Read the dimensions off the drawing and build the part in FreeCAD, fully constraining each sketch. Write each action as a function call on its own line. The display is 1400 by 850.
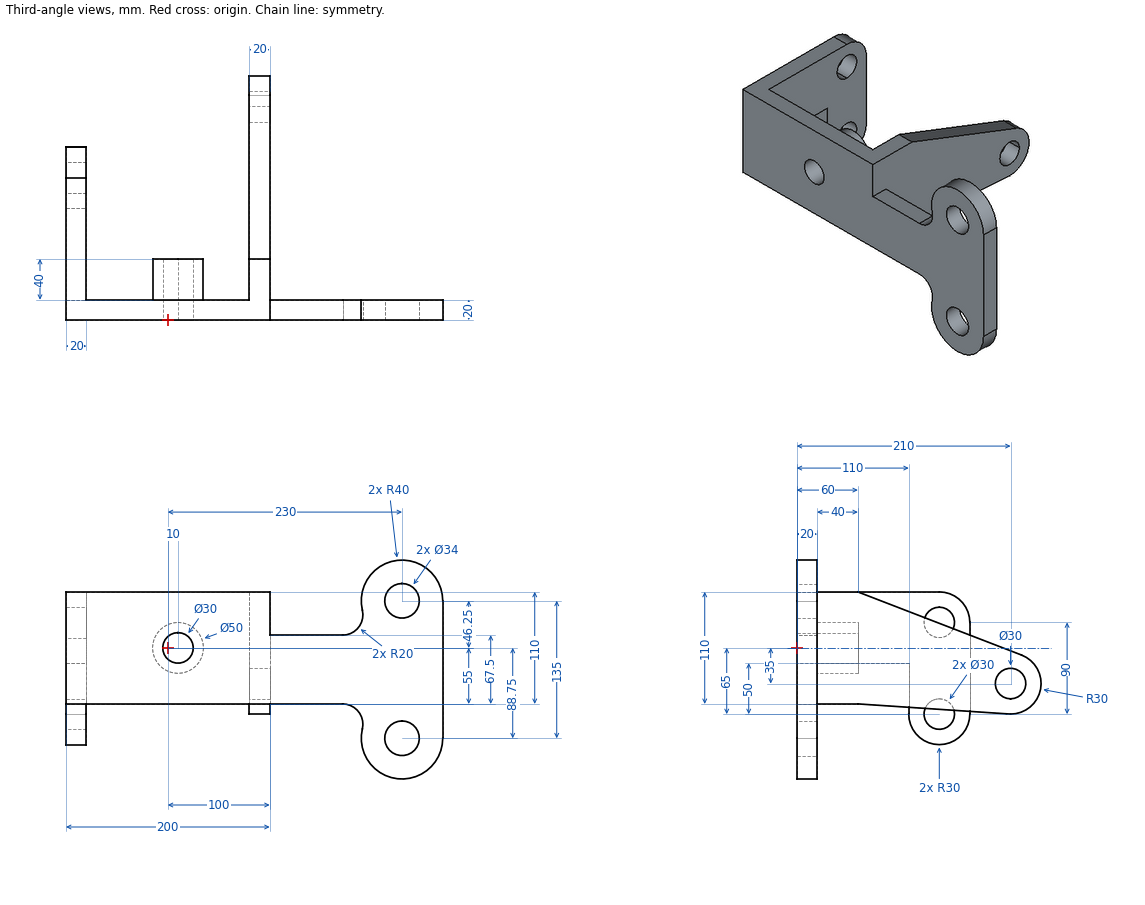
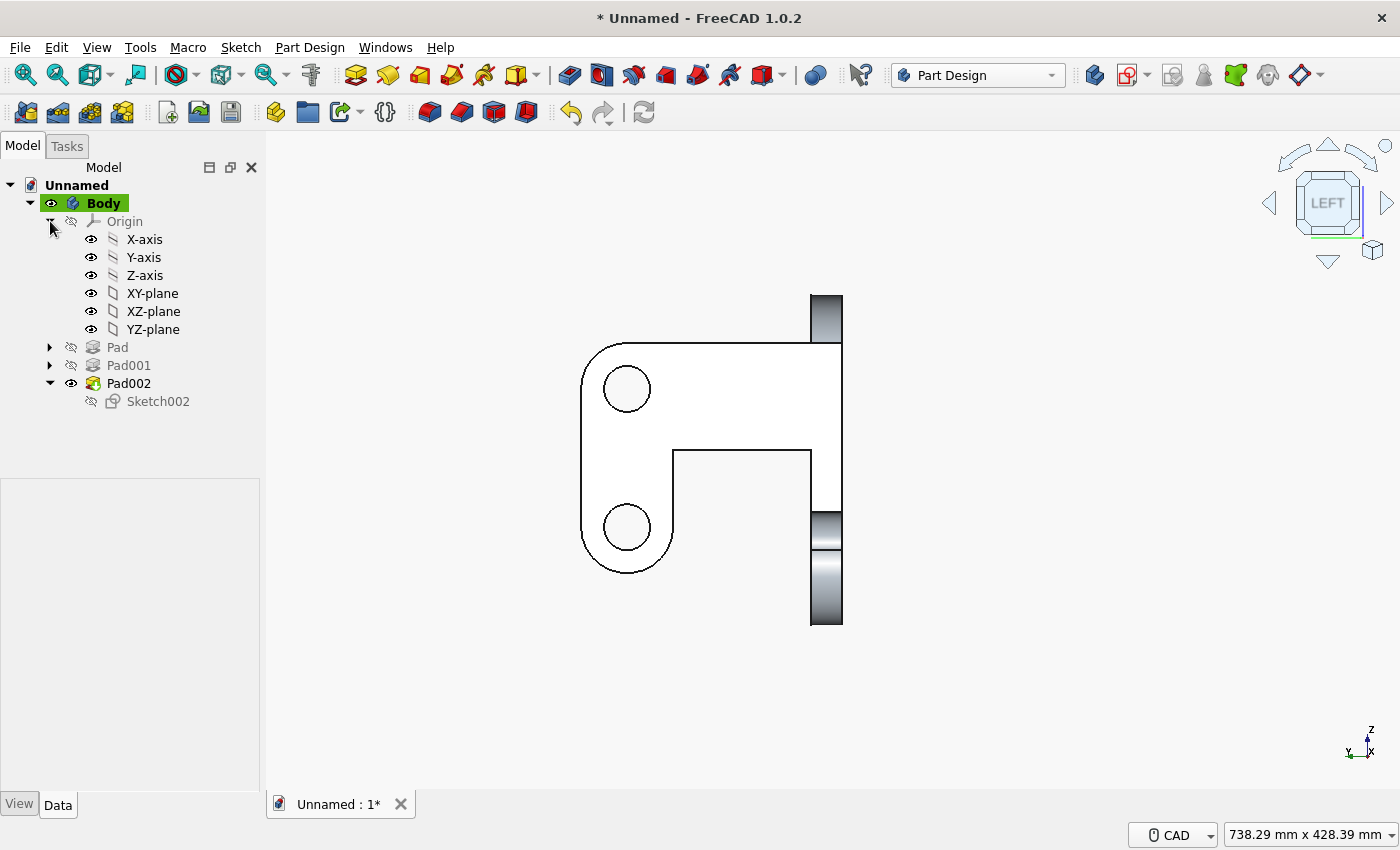
click(136, 329)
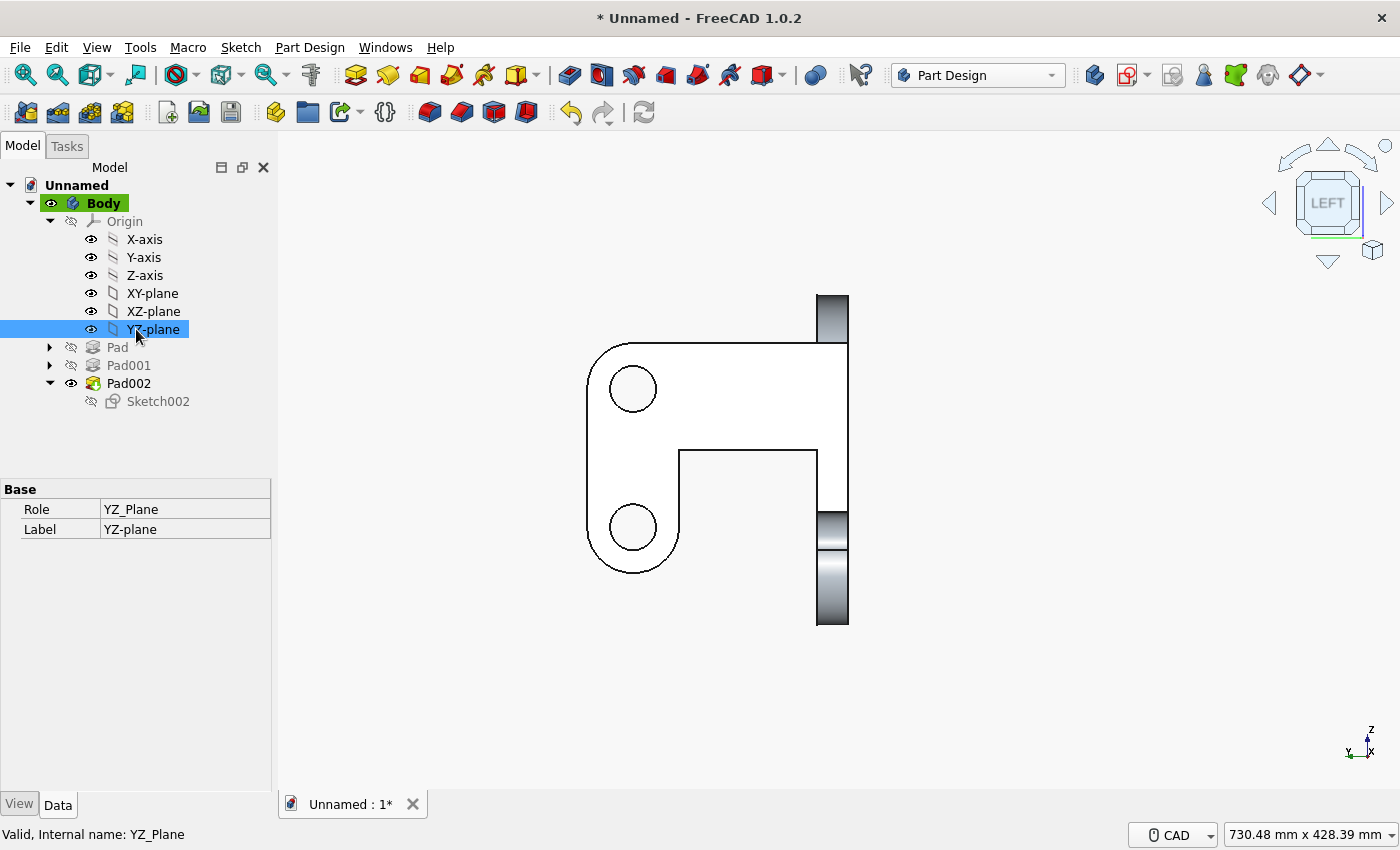
click(1300, 76)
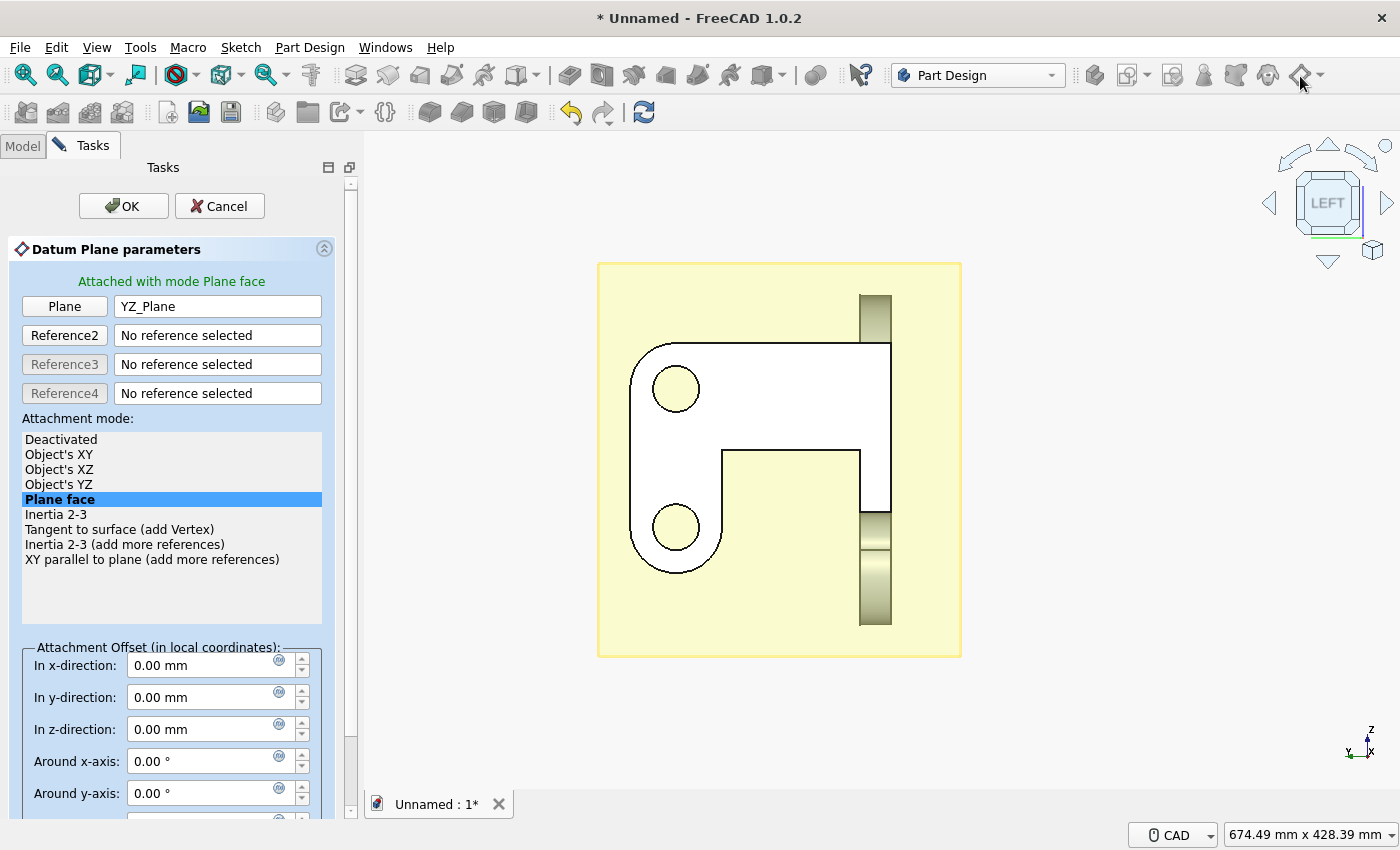
triple_click(210, 729)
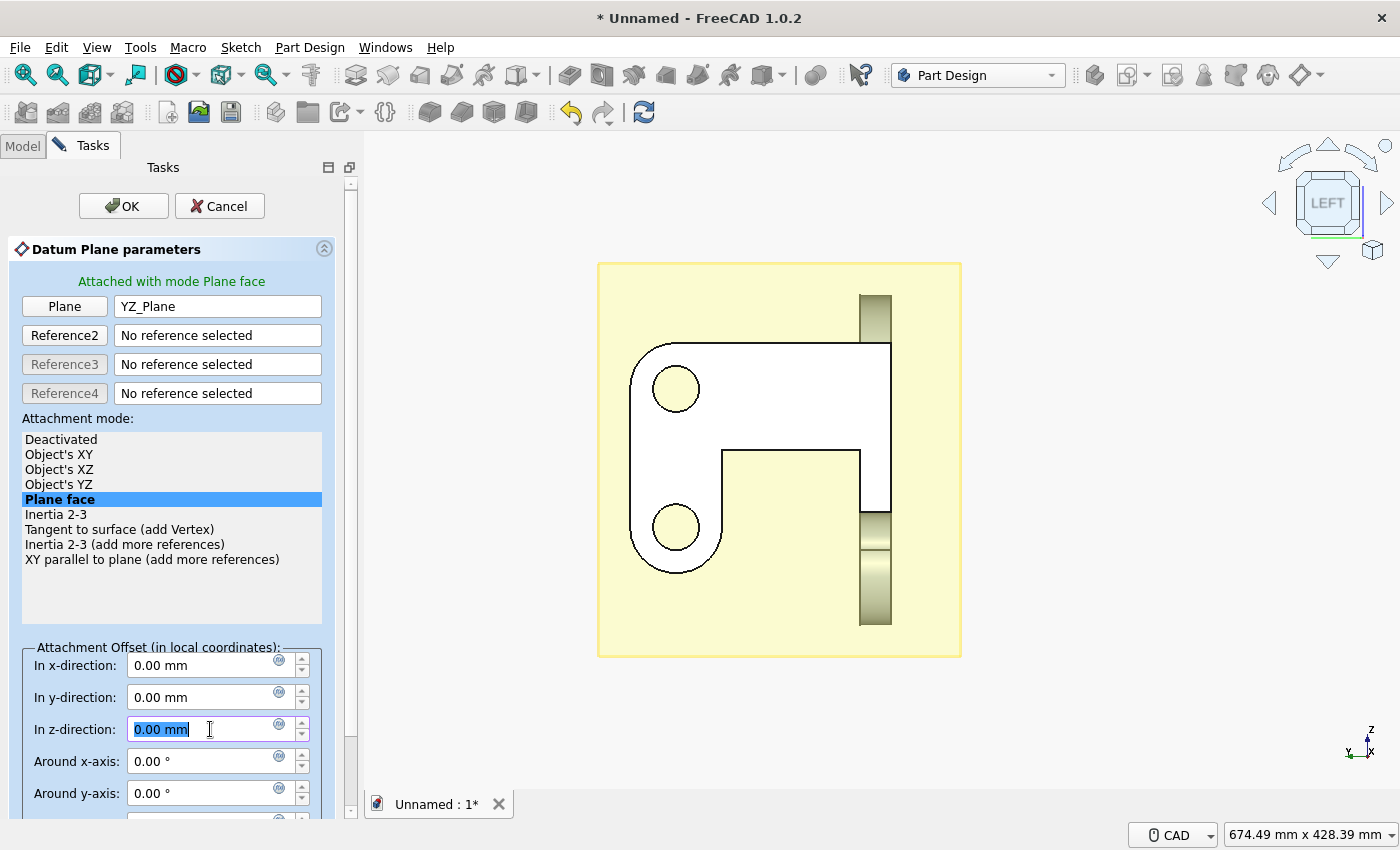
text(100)
key(Tab)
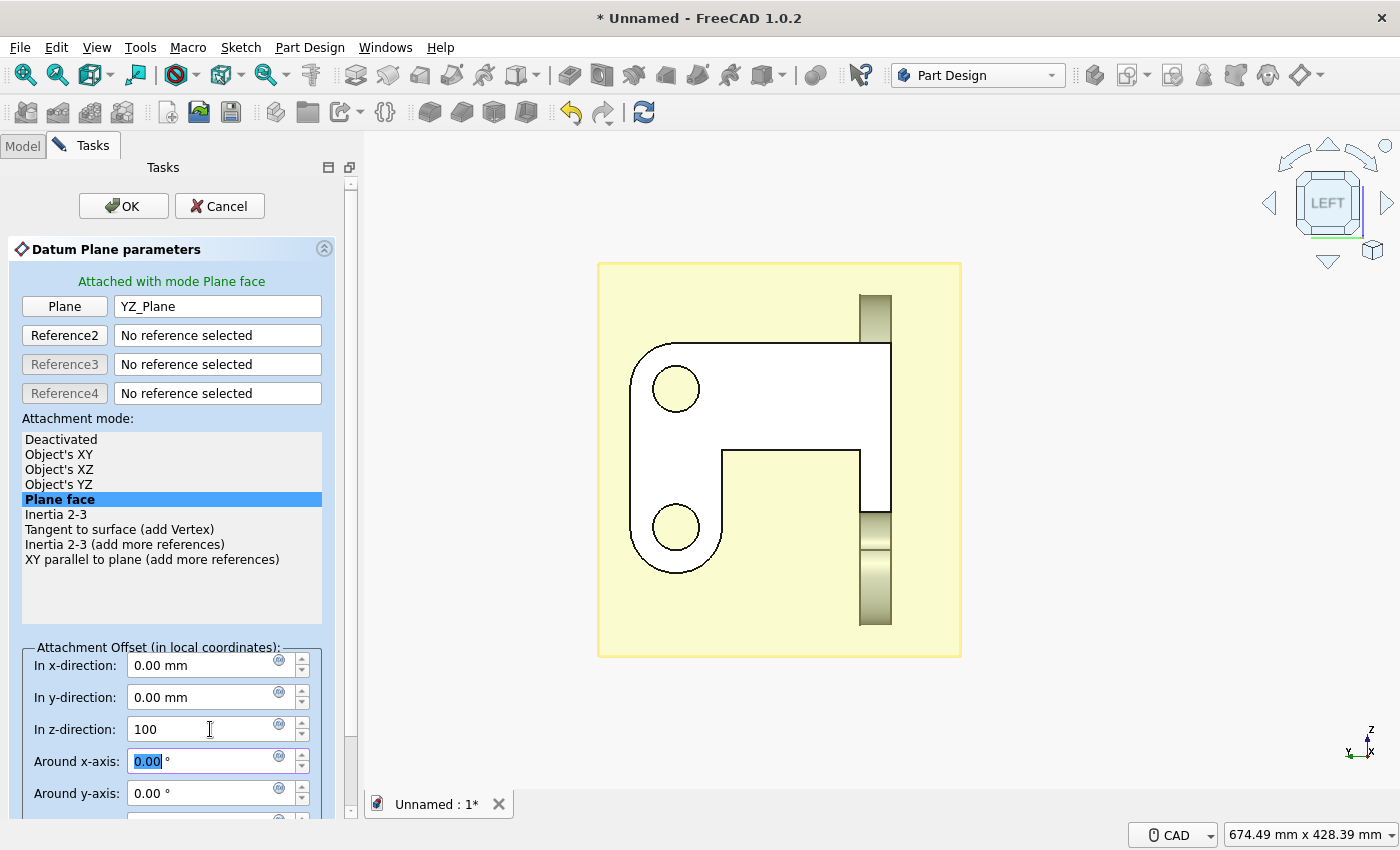
click(124, 206)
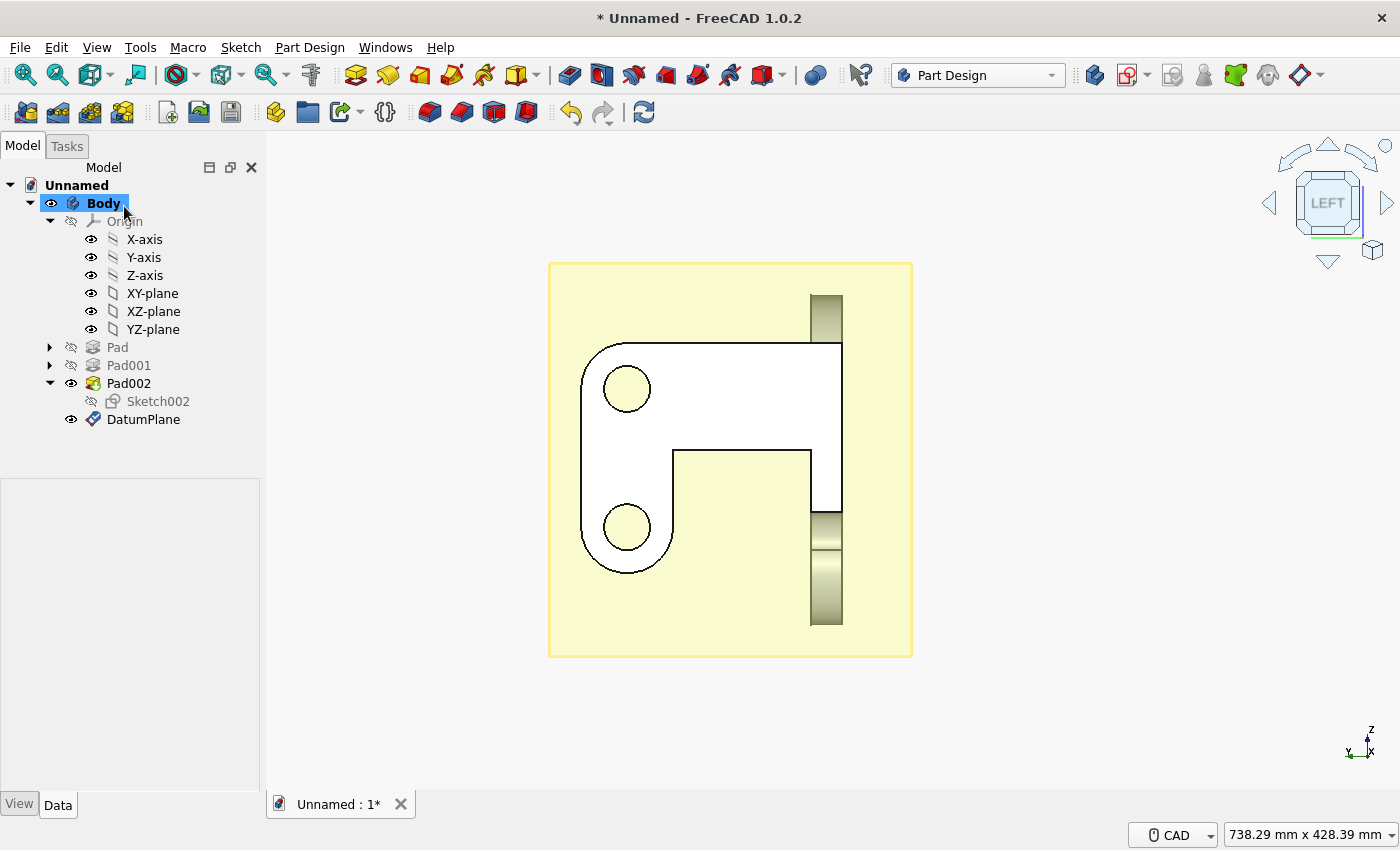
click(116, 419)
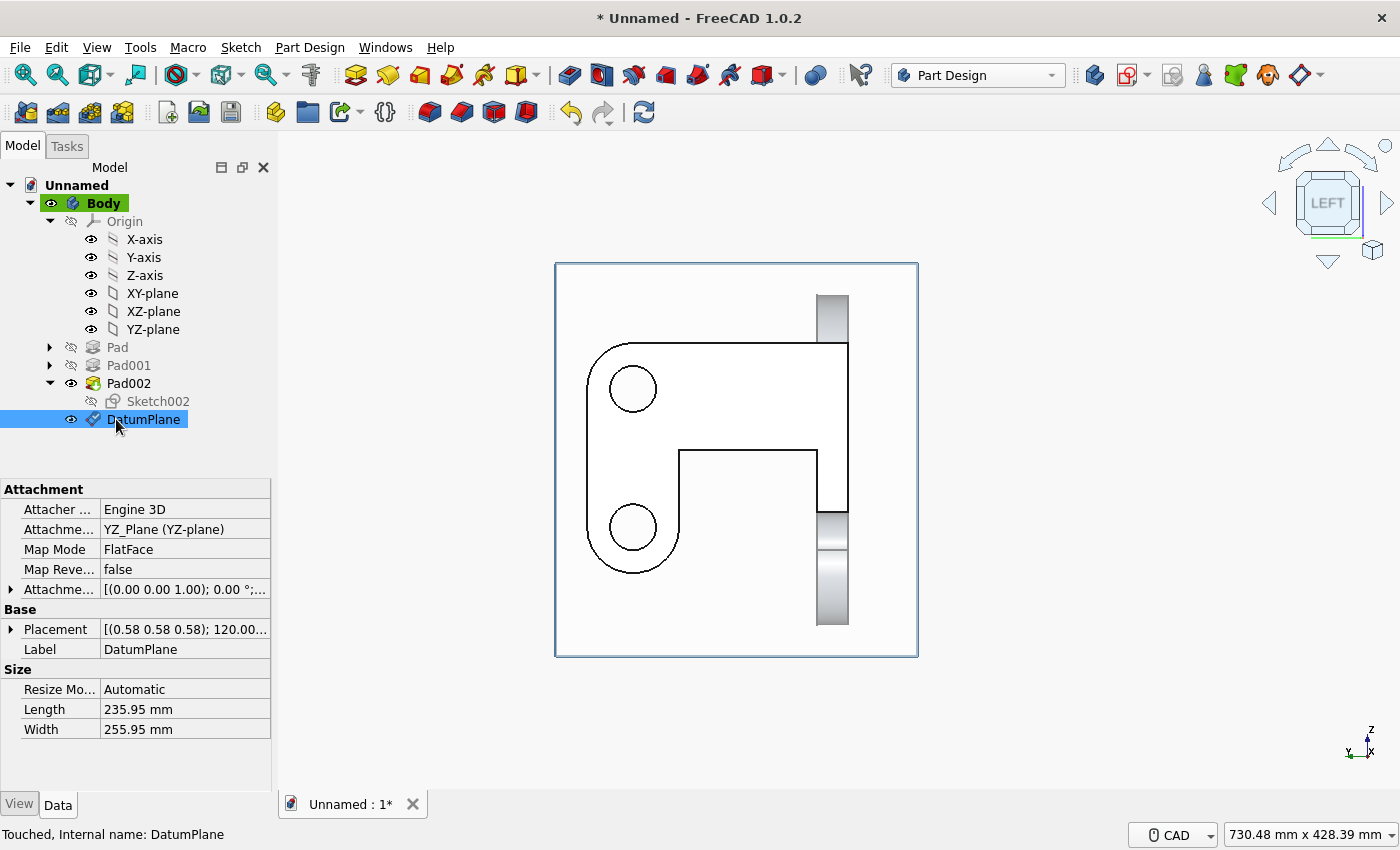
click(1128, 76)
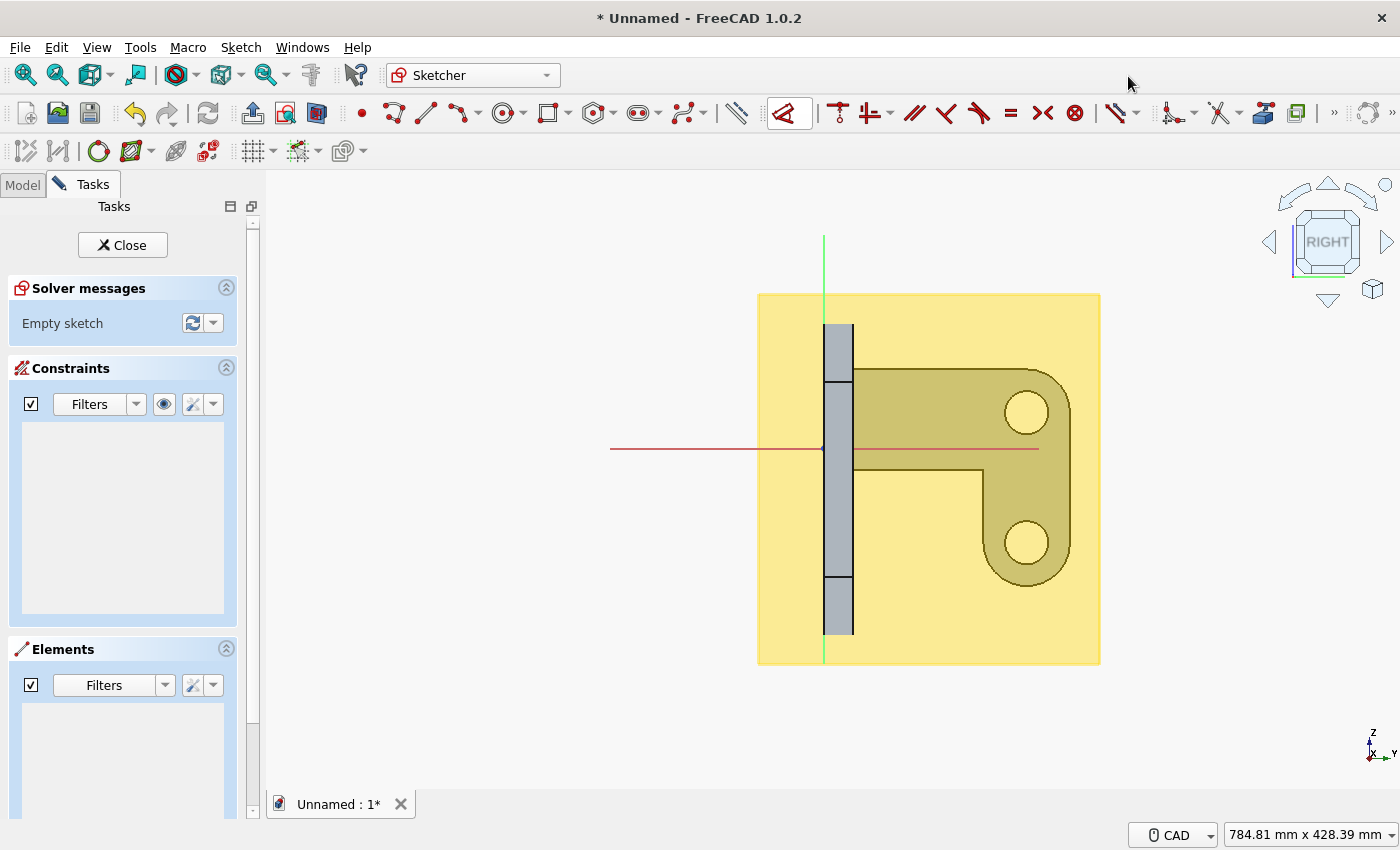
key(q)
key(s)